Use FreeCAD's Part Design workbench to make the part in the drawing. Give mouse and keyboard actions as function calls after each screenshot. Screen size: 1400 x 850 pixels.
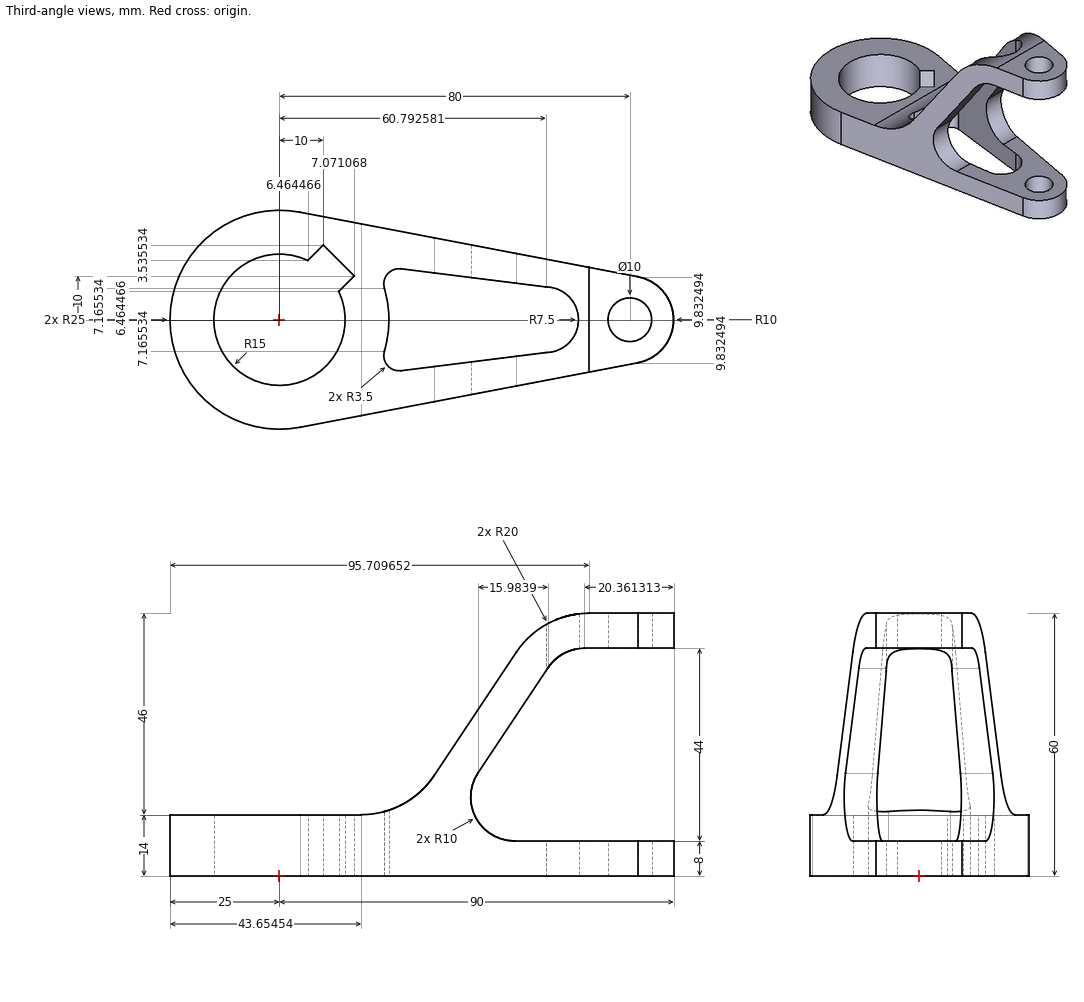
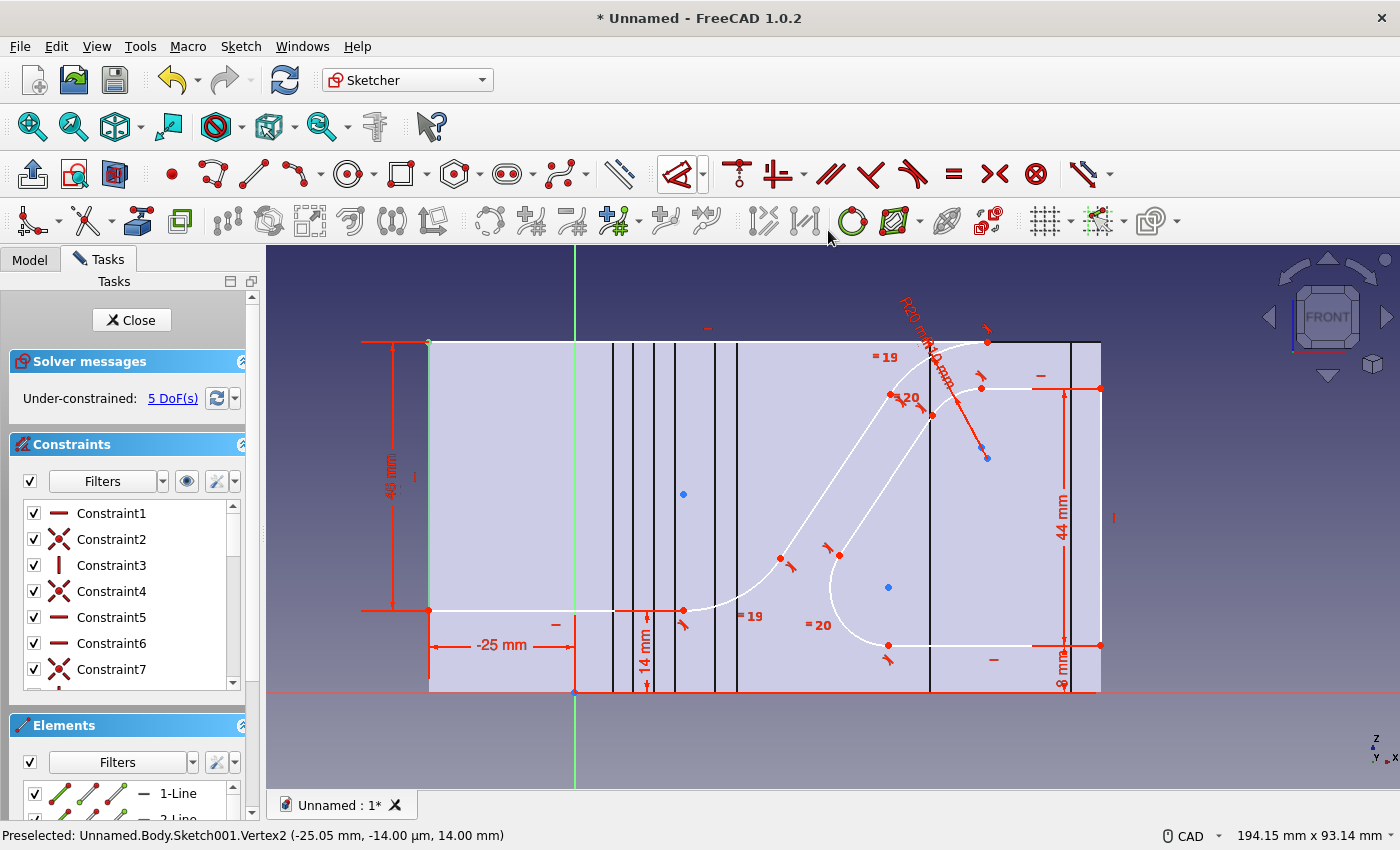
click(1101, 389)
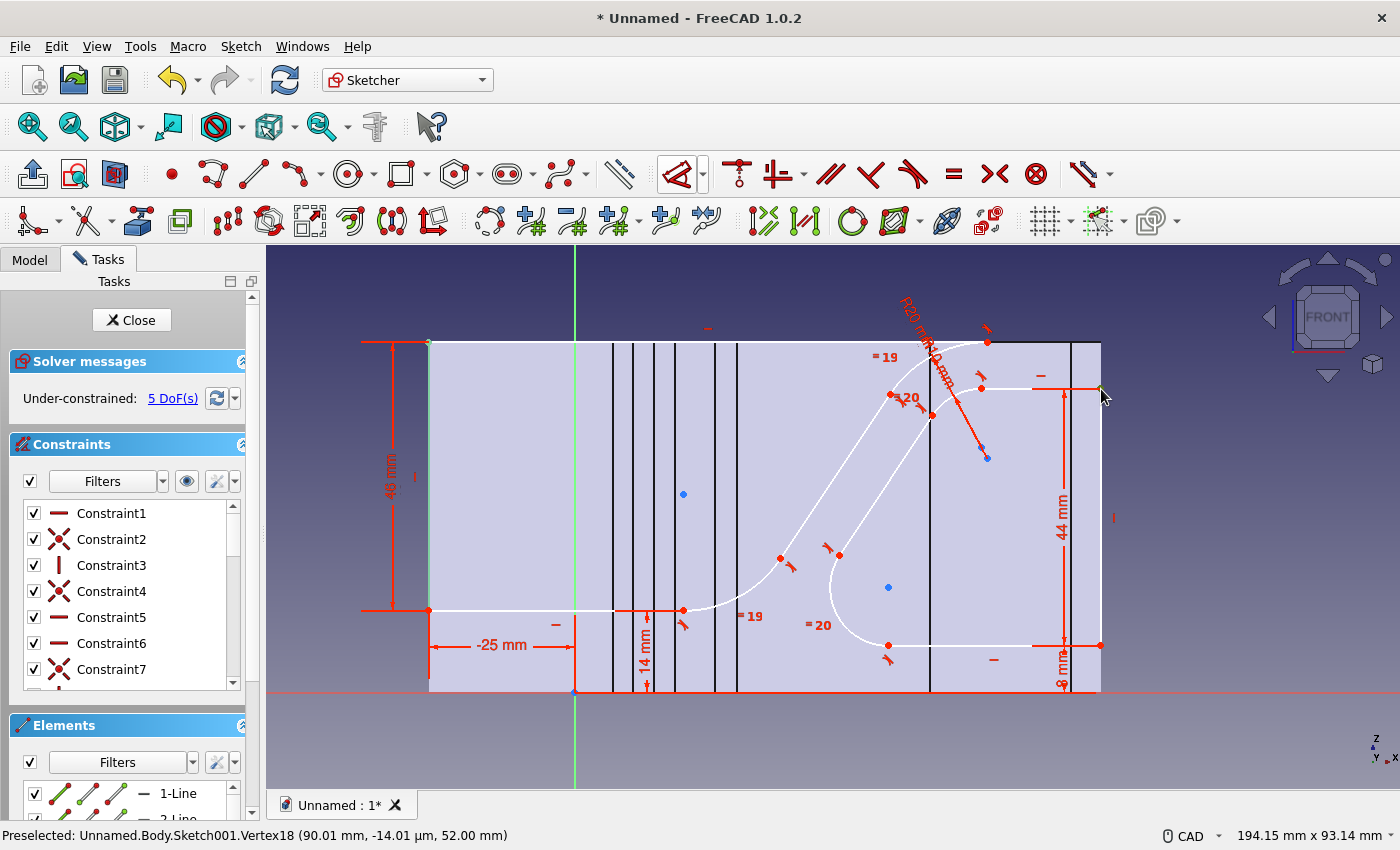
key(l)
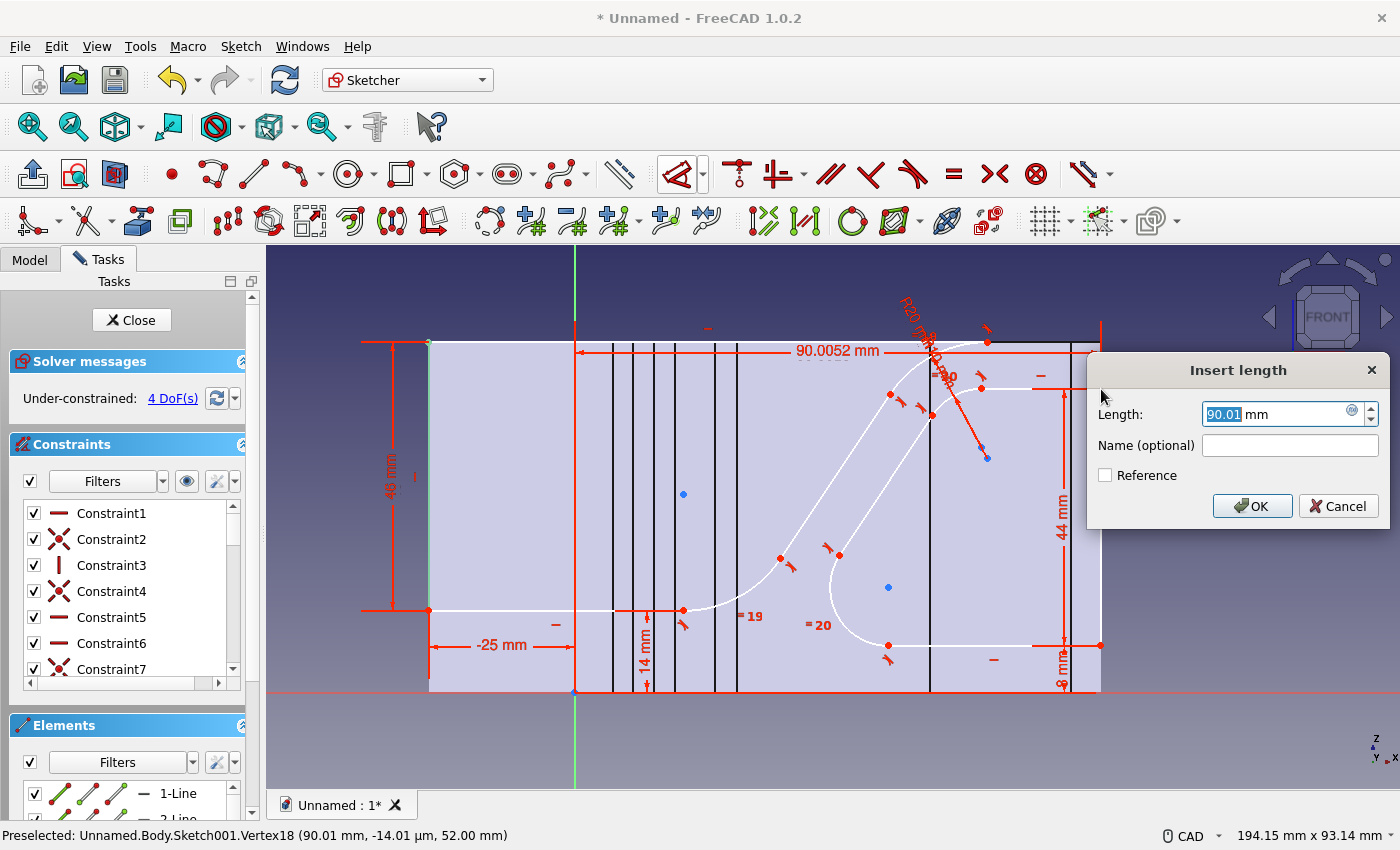
text(90)
key(Return)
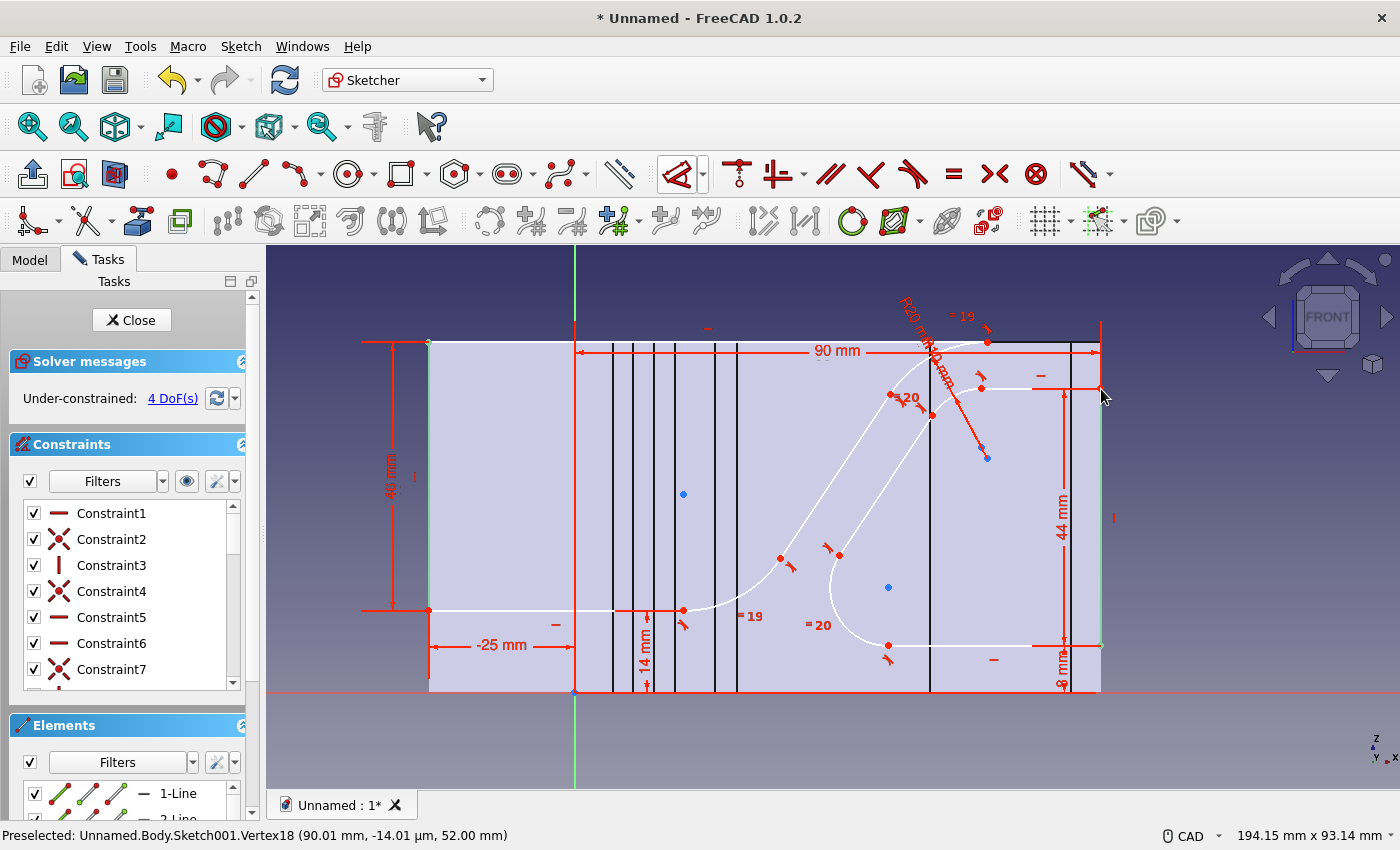
click(607, 611)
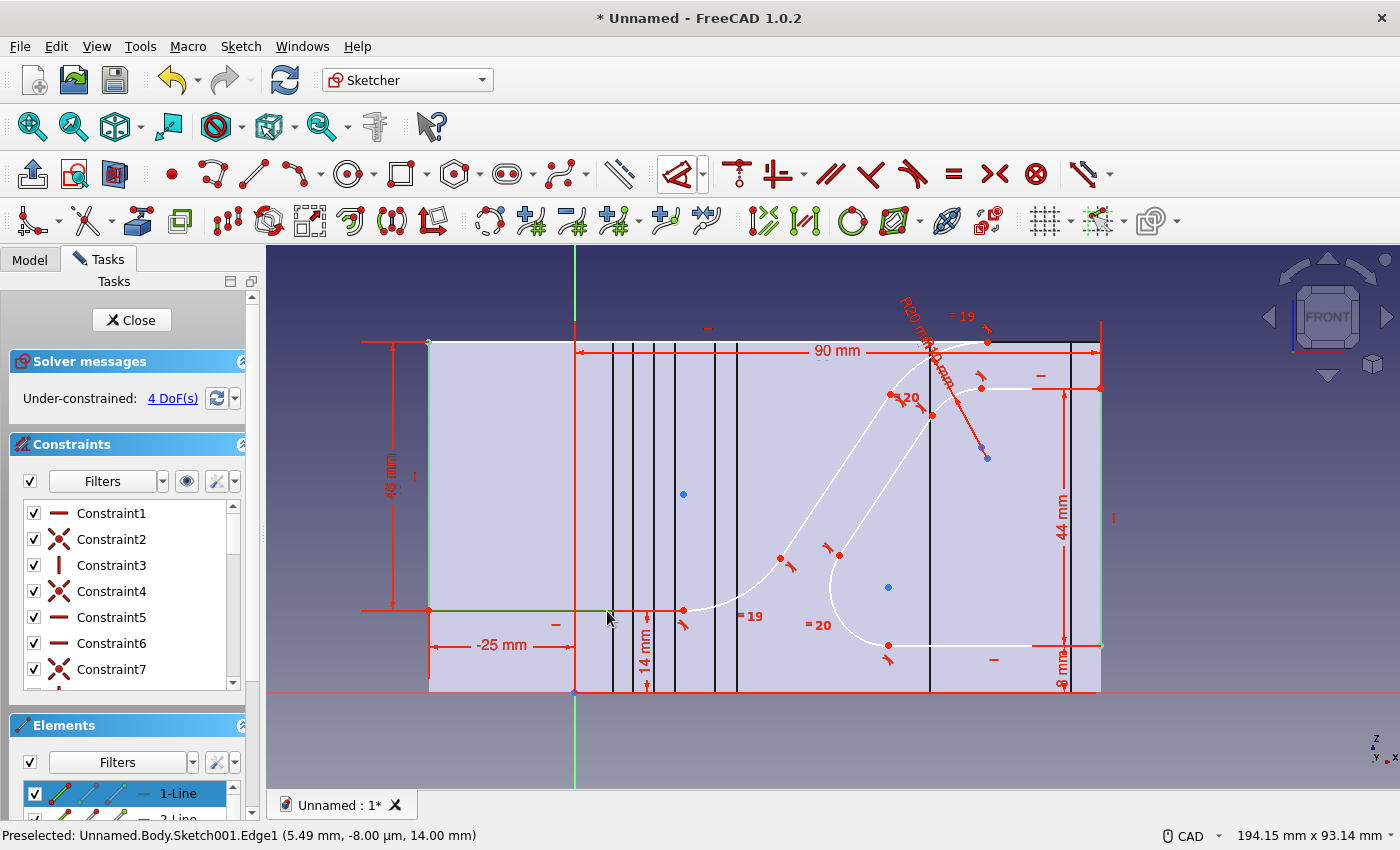
click(702, 174)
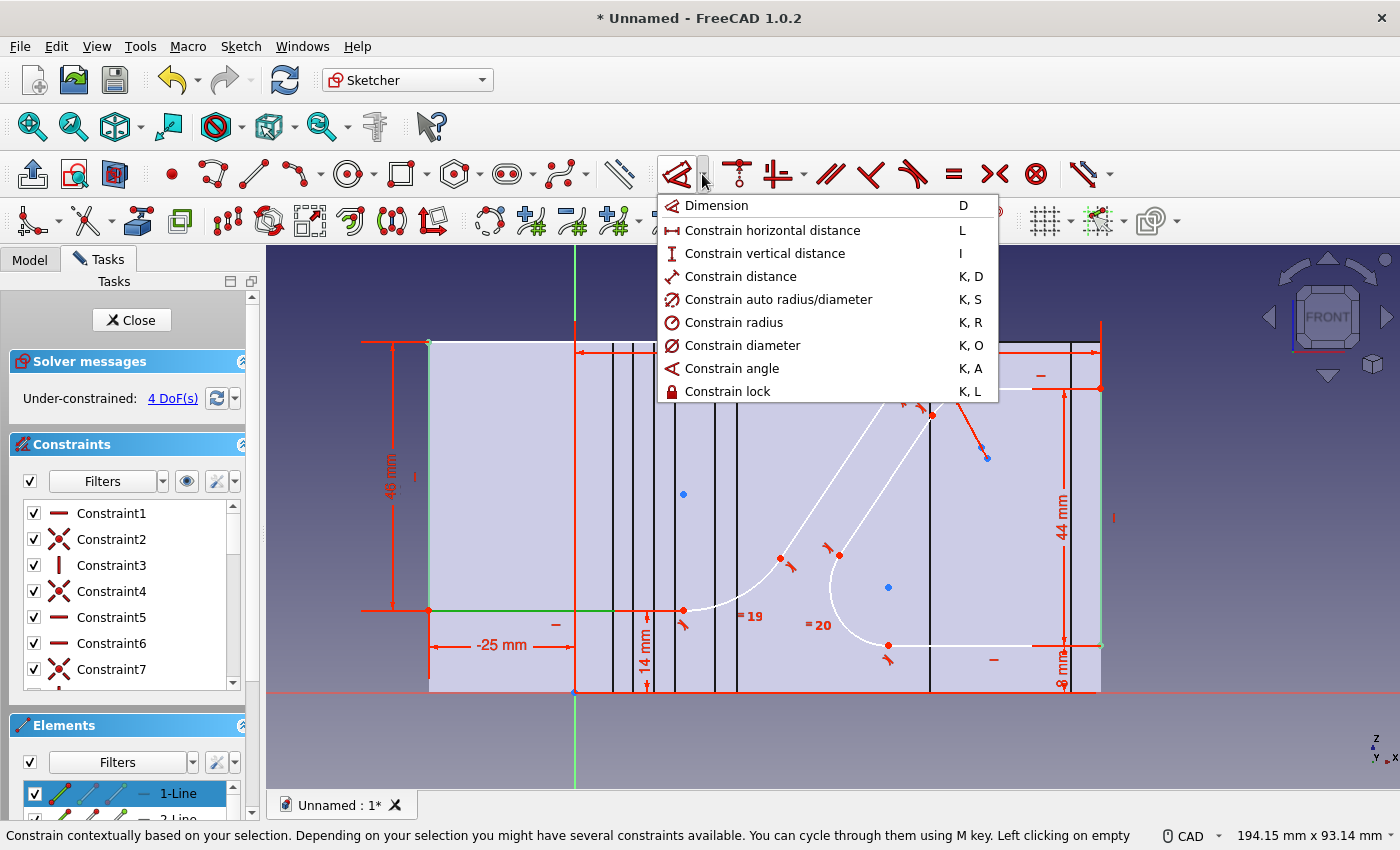
click(828, 230)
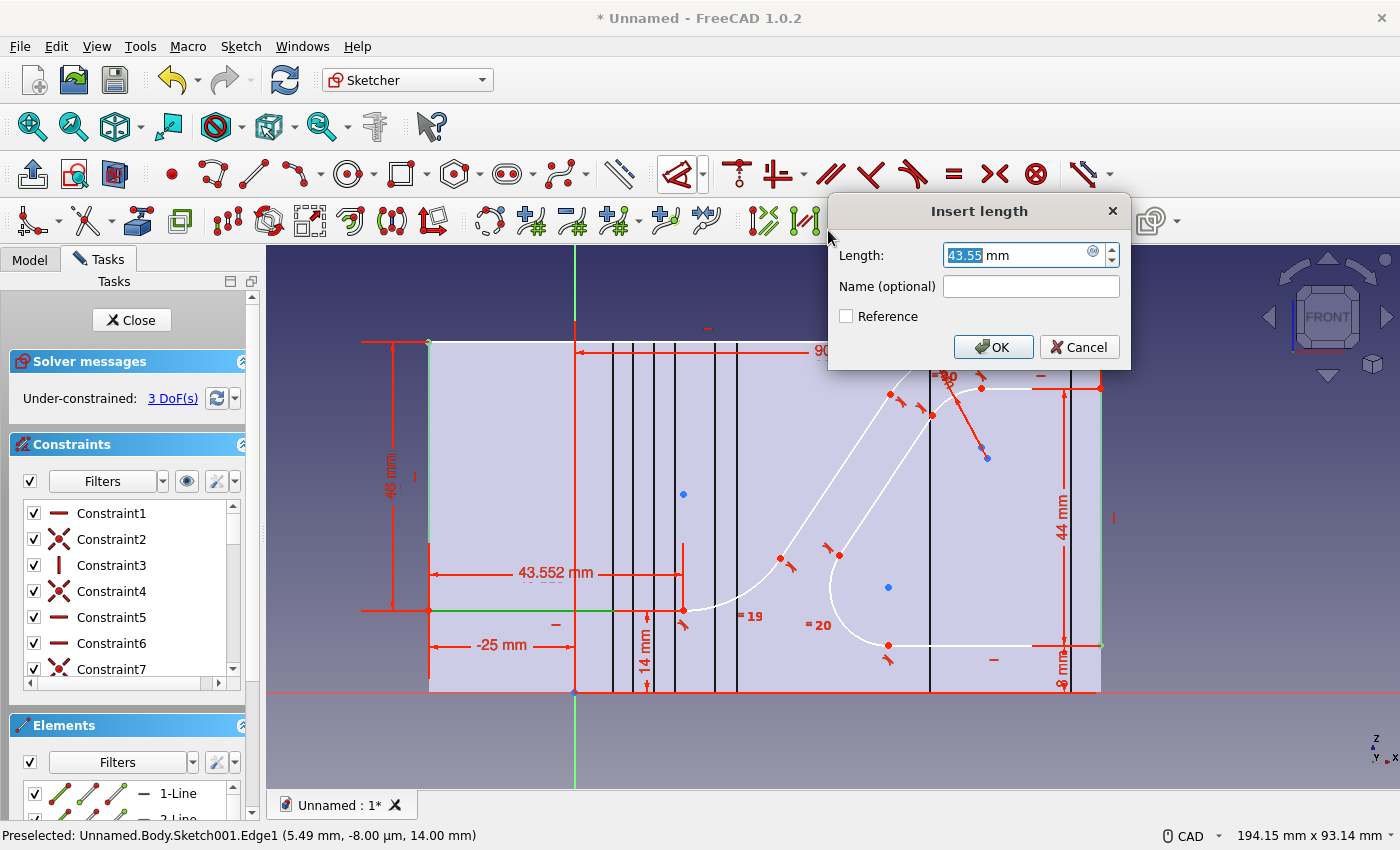
text(43.65454)
key(Return)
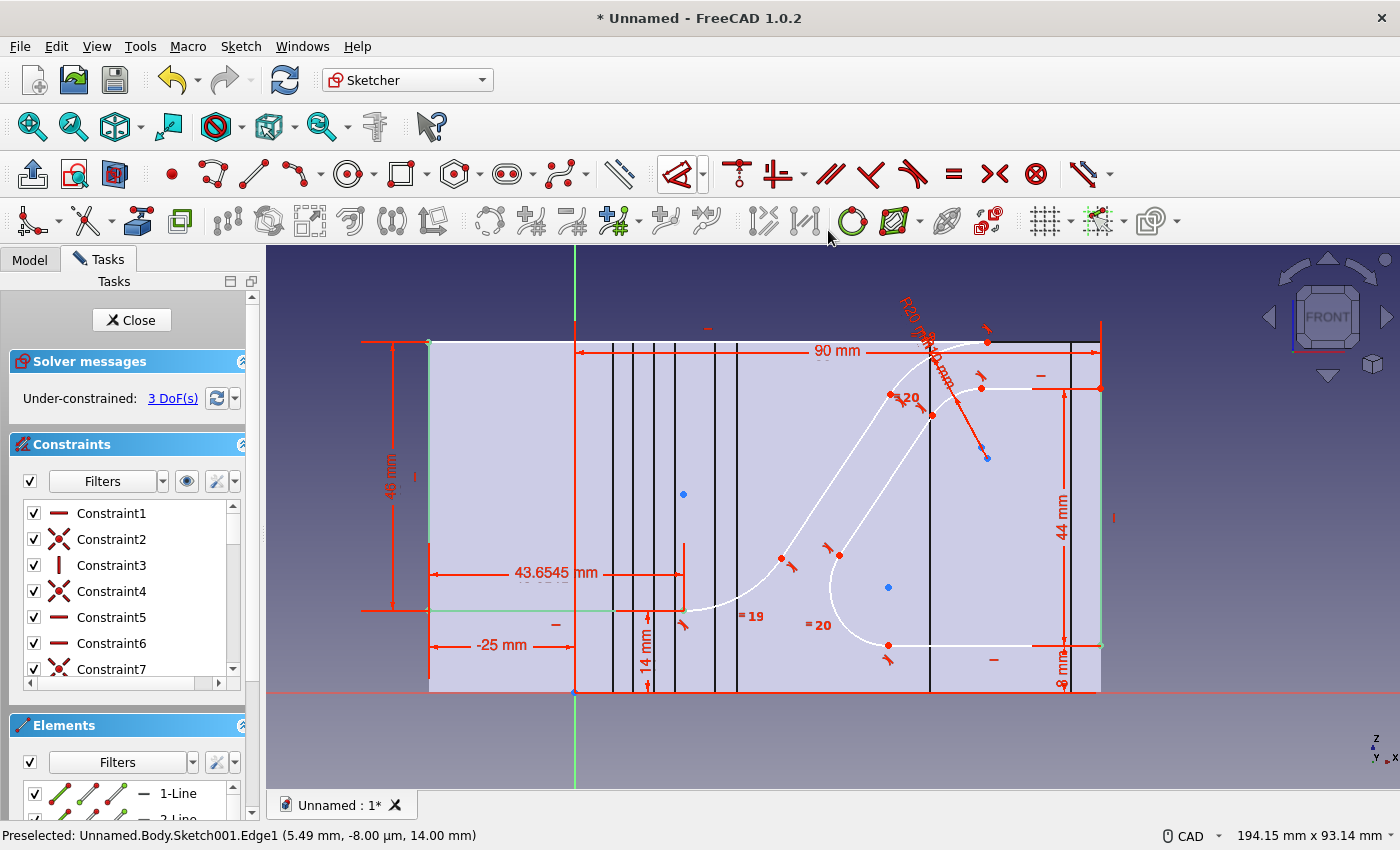
click(868, 513)